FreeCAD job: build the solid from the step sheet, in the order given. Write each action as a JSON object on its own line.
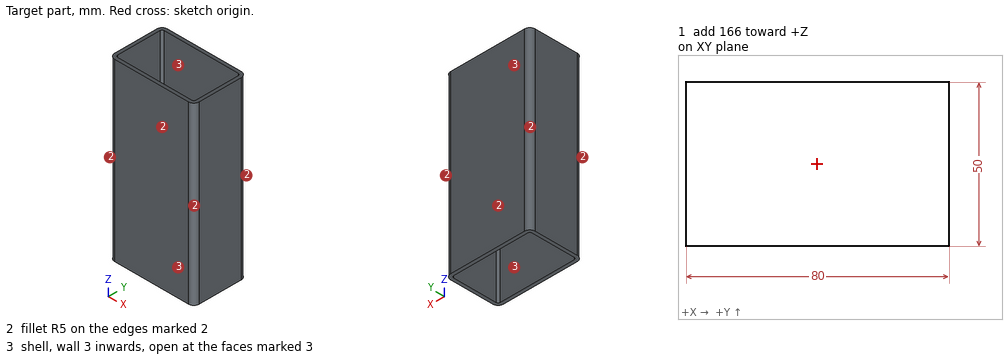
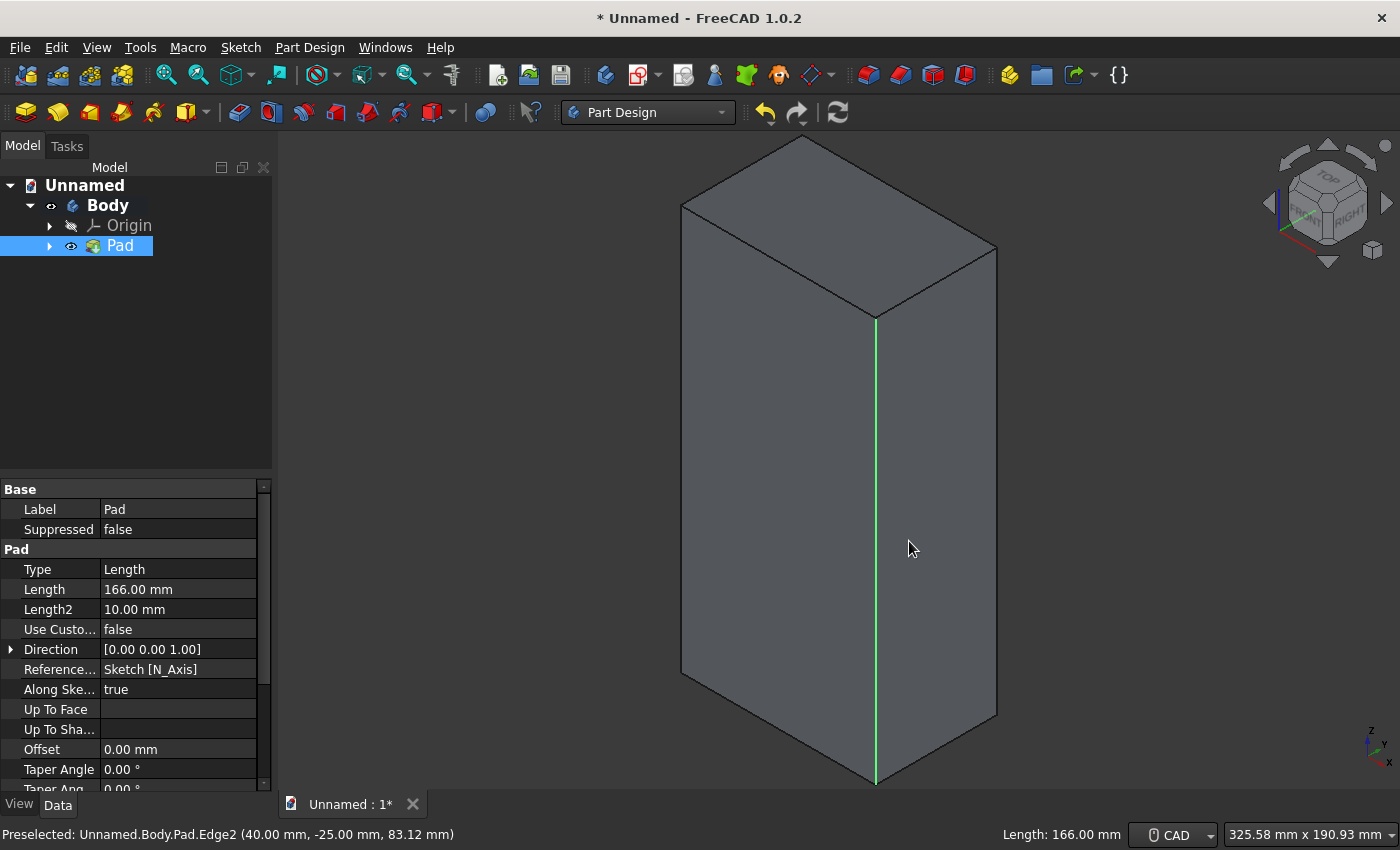
{"action": "key", "text": "2"}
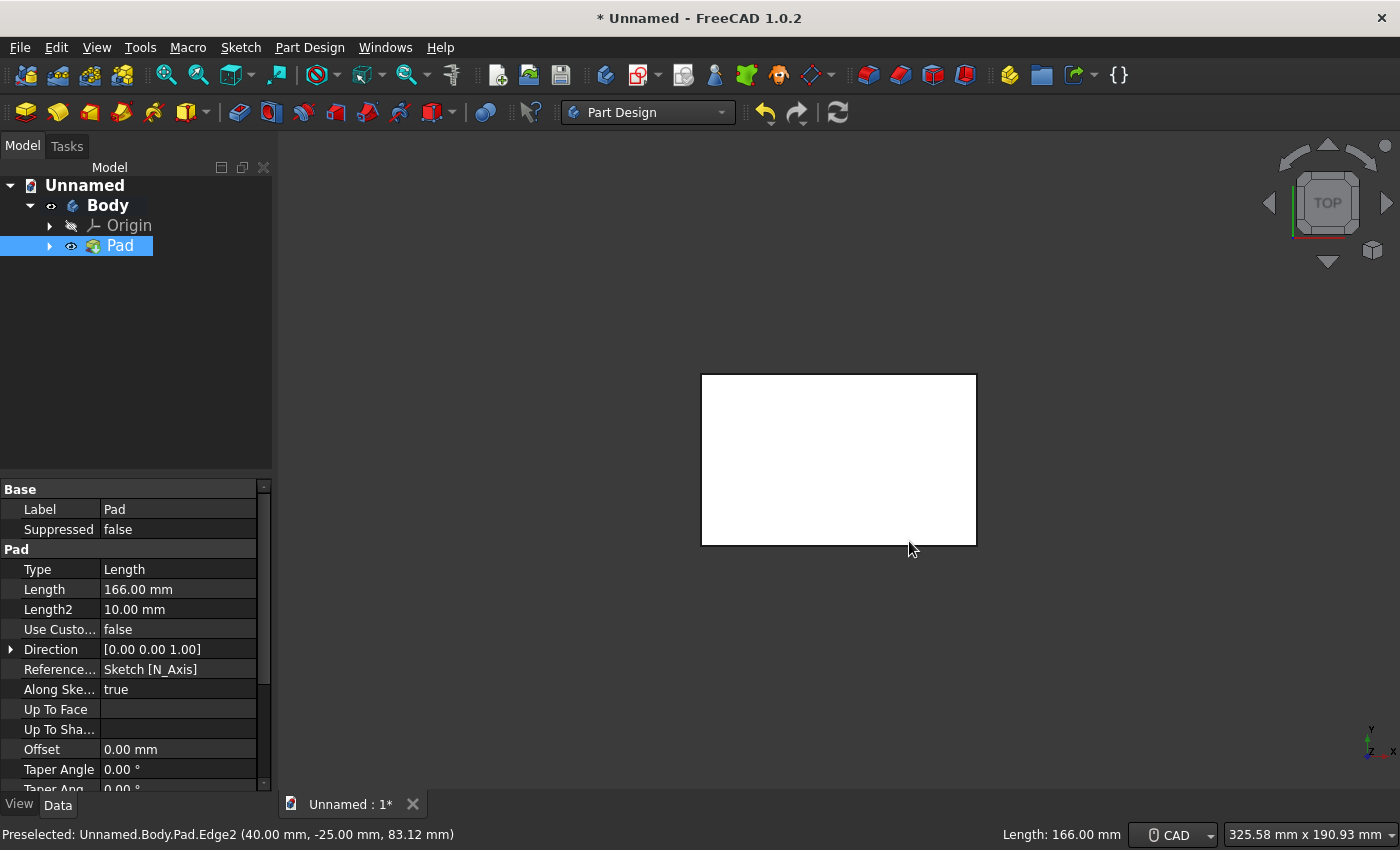
{"action": "key", "text": "v f"}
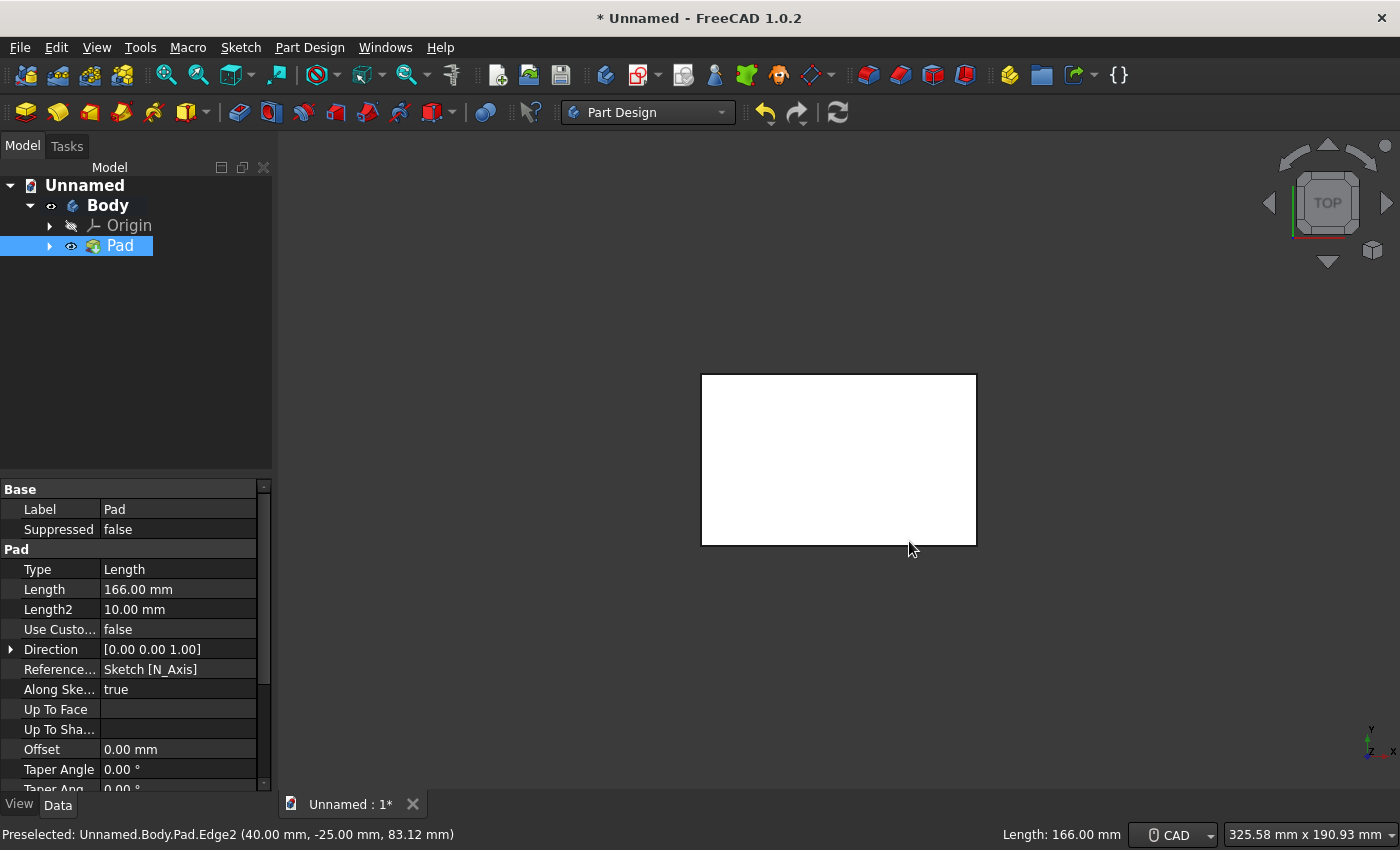
{"action": "key", "text": "1"}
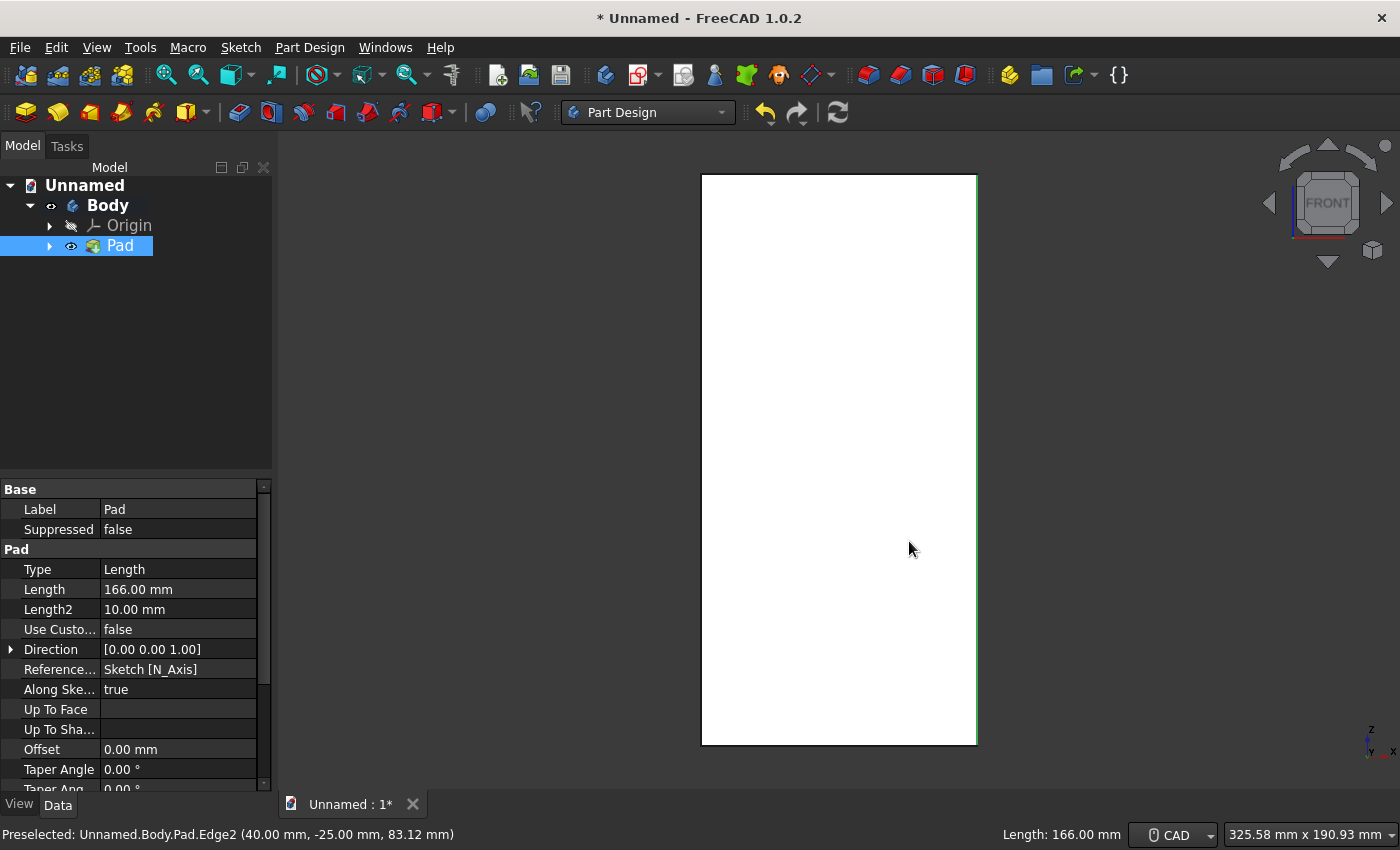
{"action": "left_click", "coordinate": [701, 459], "text": "ctrl"}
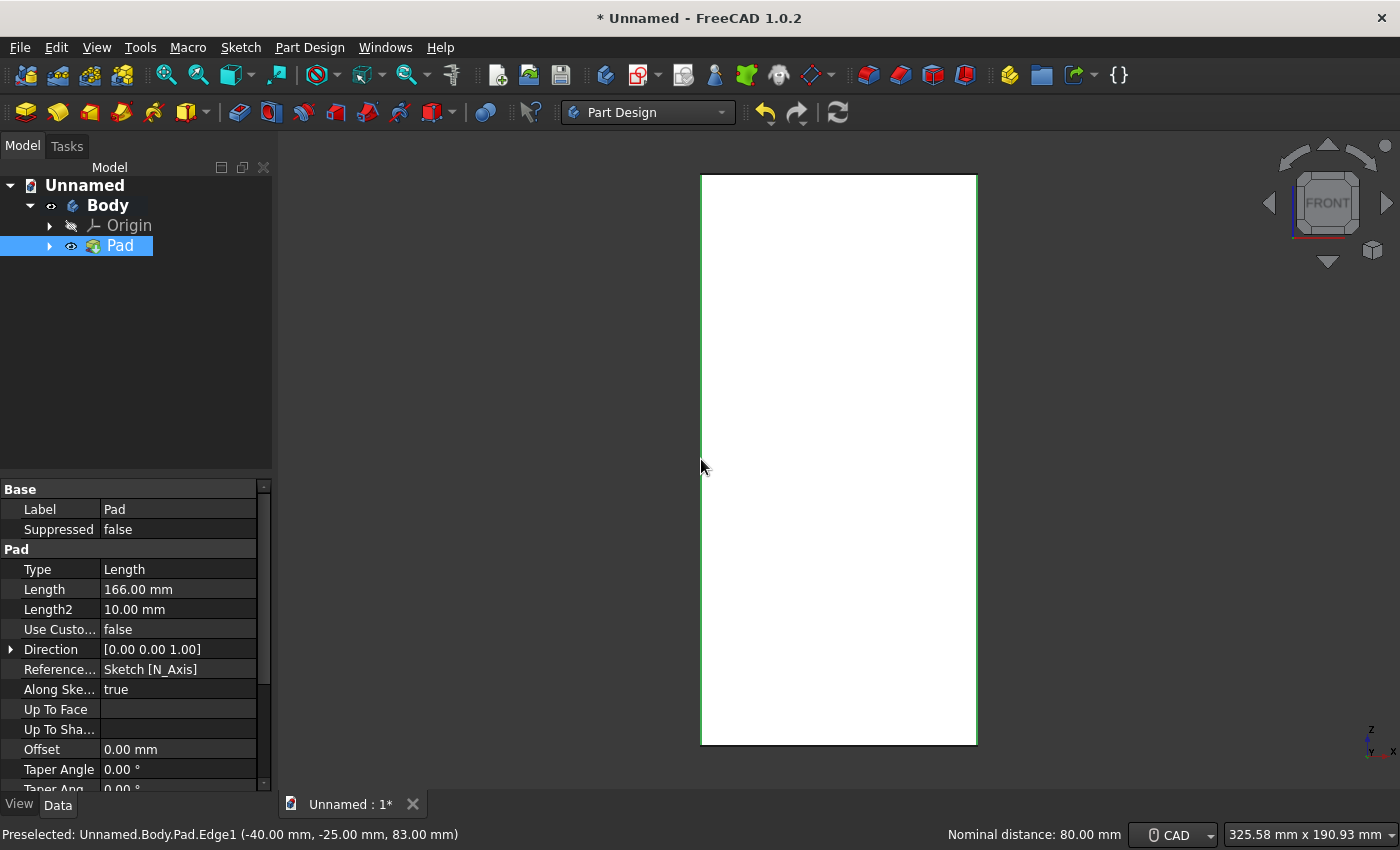
{"action": "key", "text": "3"}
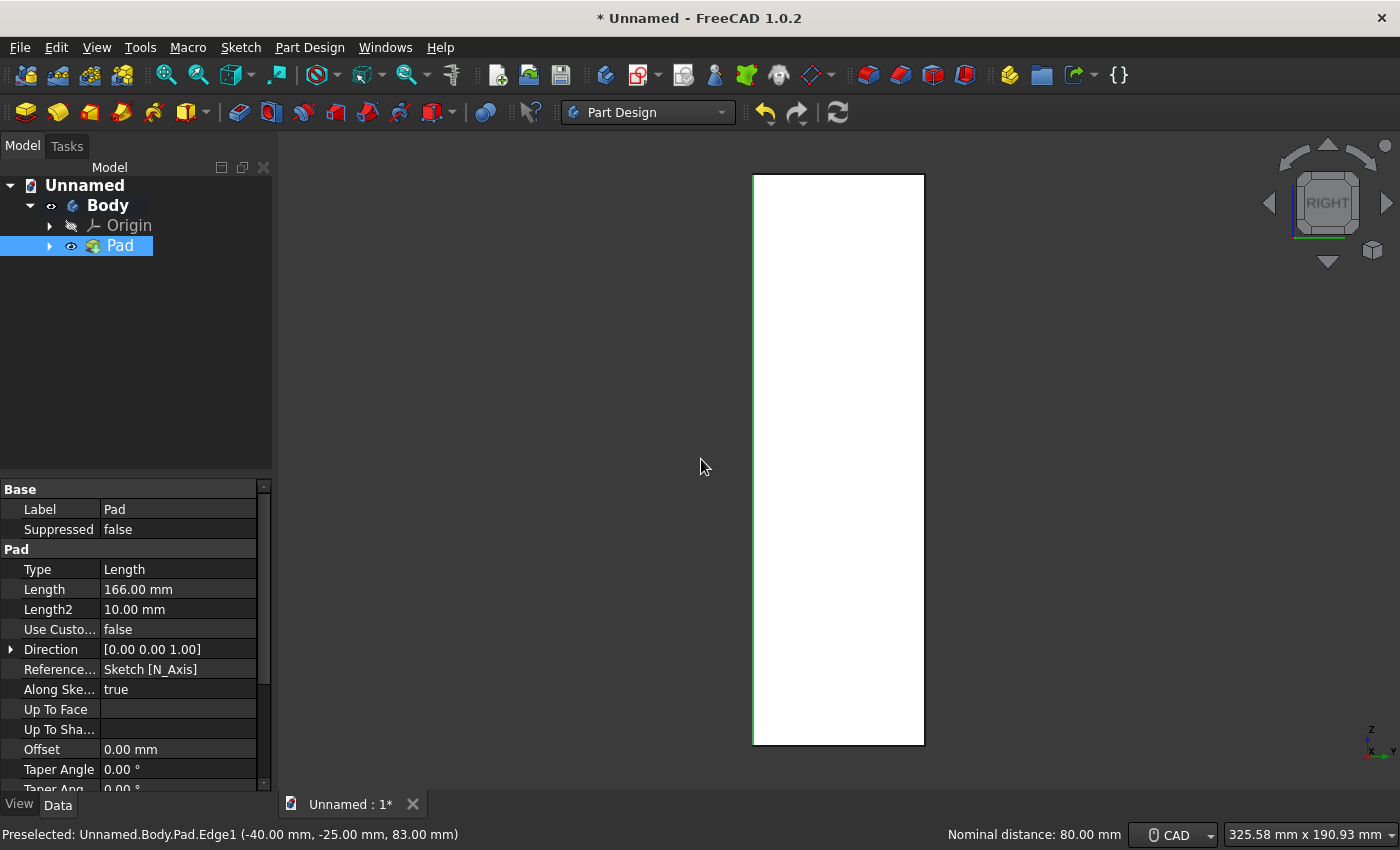
{"action": "left_click", "coordinate": [925, 459], "text": "ctrl"}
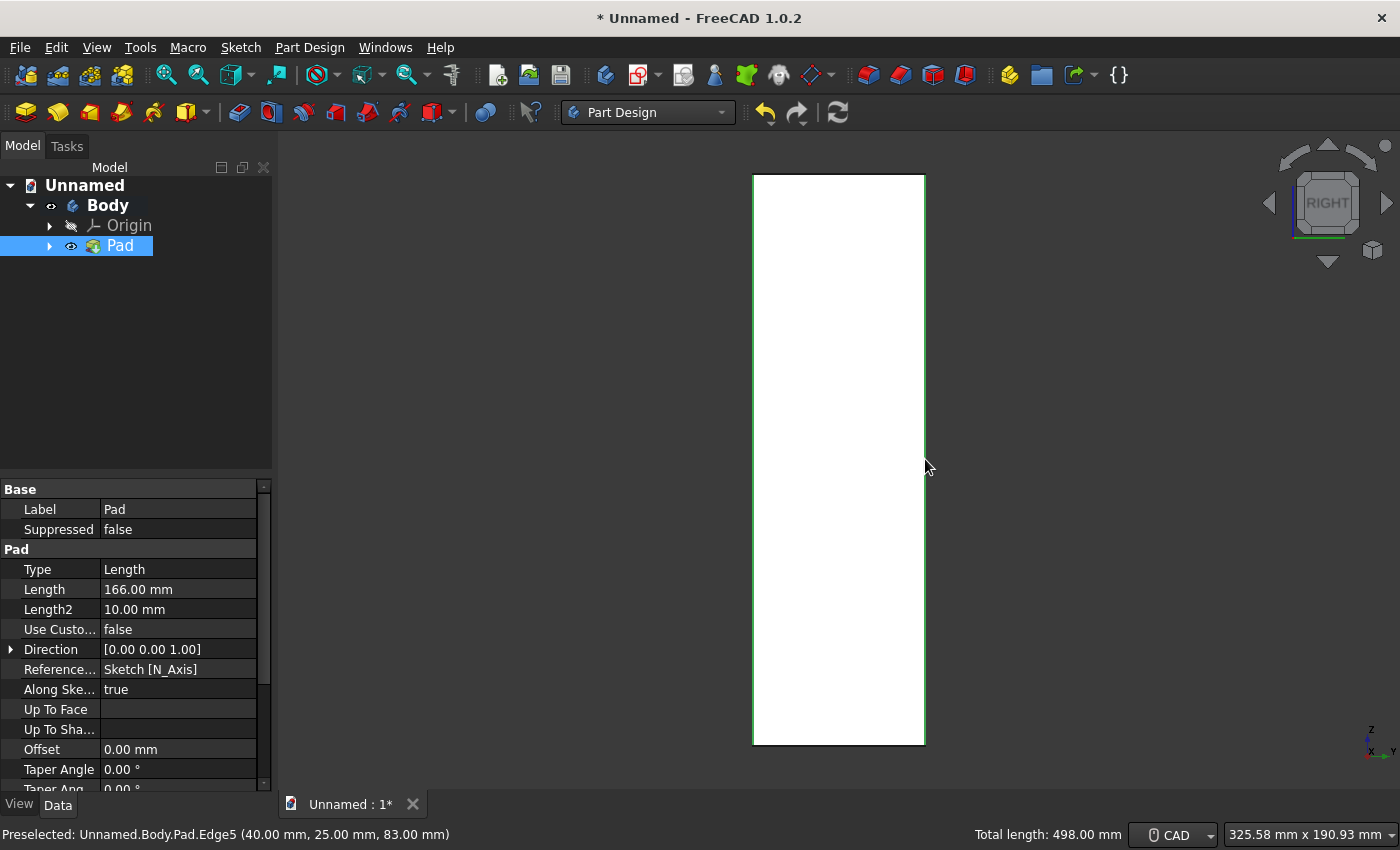
{"action": "key", "text": "5"}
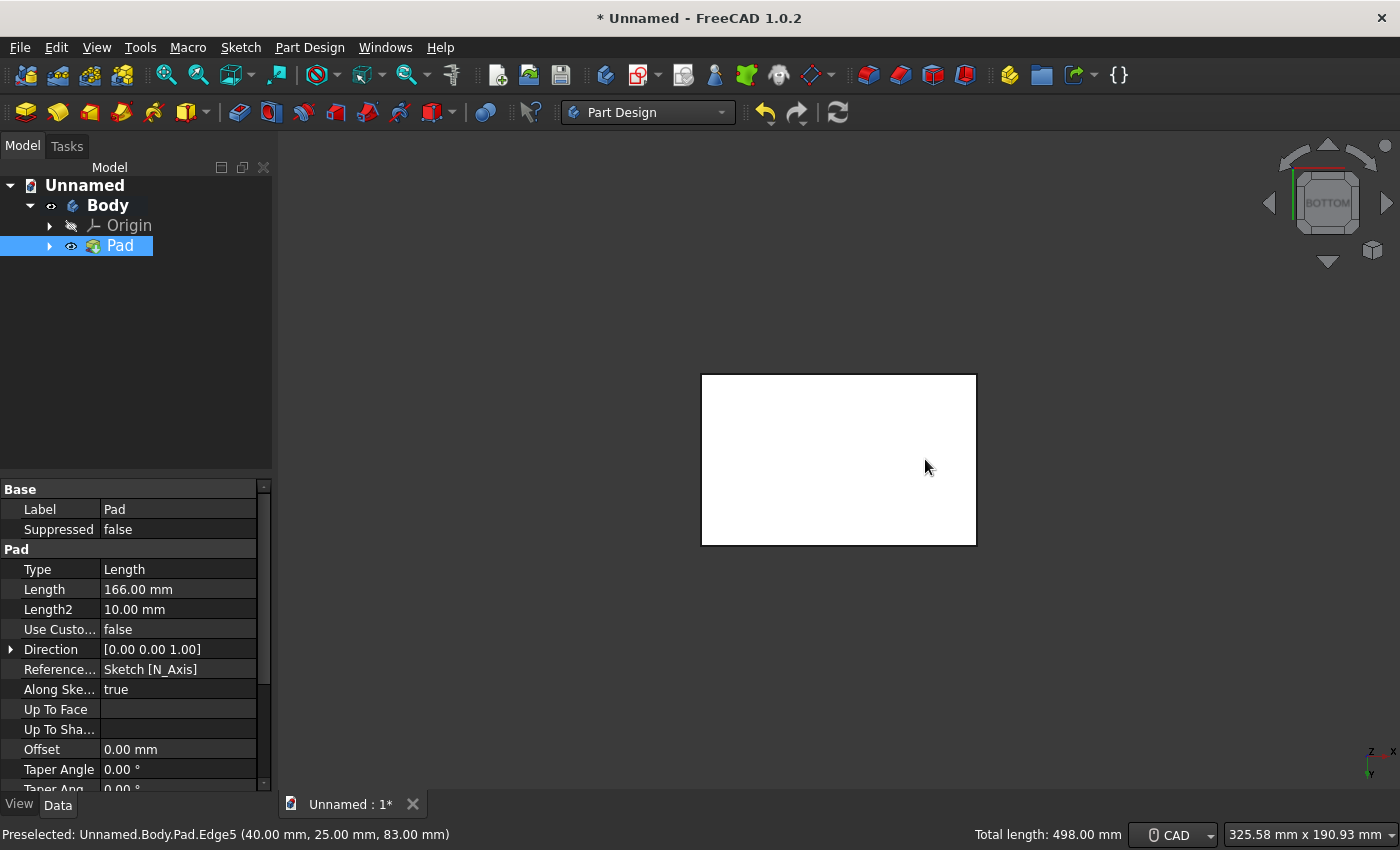
{"action": "key", "text": "v f"}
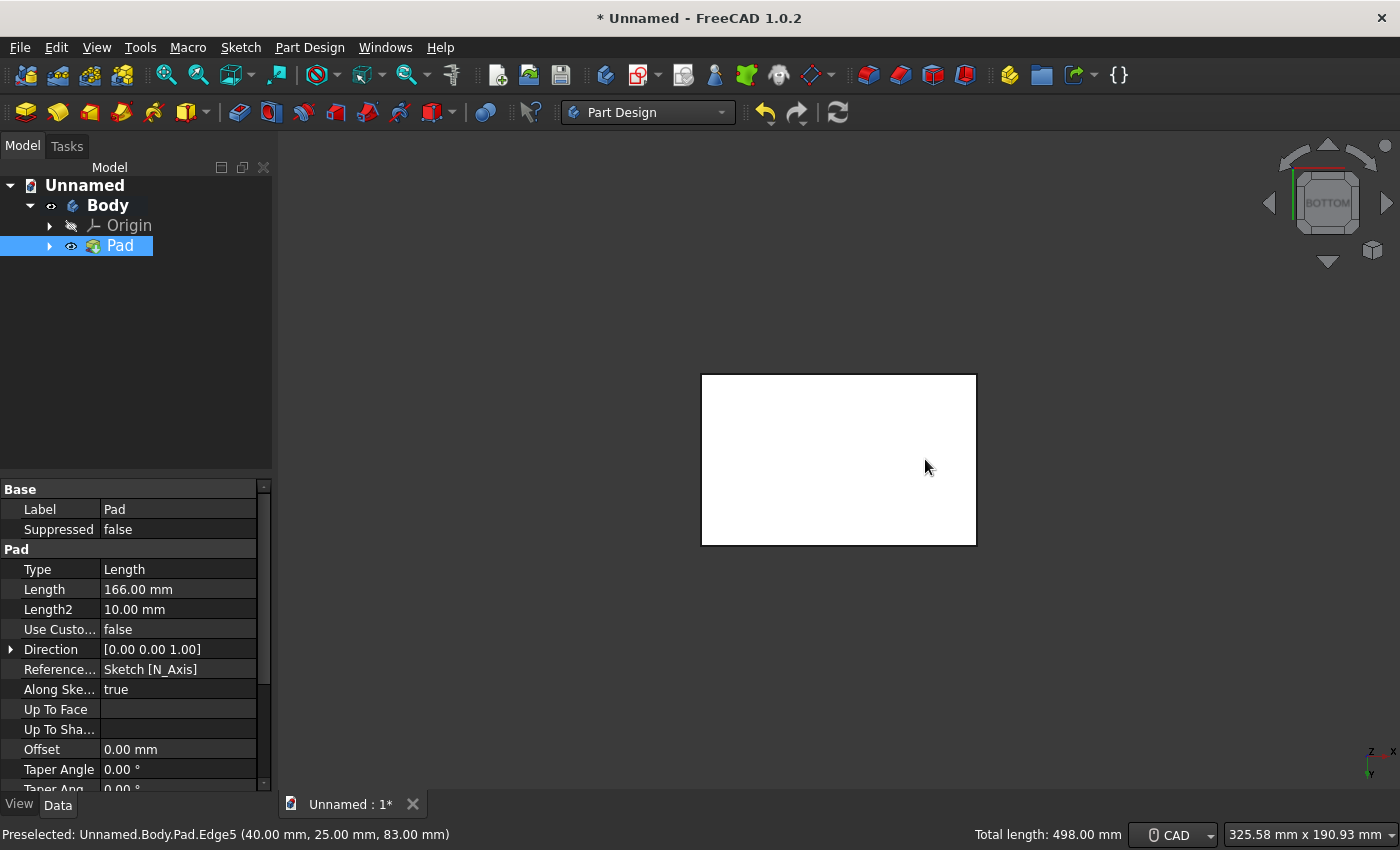
{"action": "key", "text": "4"}